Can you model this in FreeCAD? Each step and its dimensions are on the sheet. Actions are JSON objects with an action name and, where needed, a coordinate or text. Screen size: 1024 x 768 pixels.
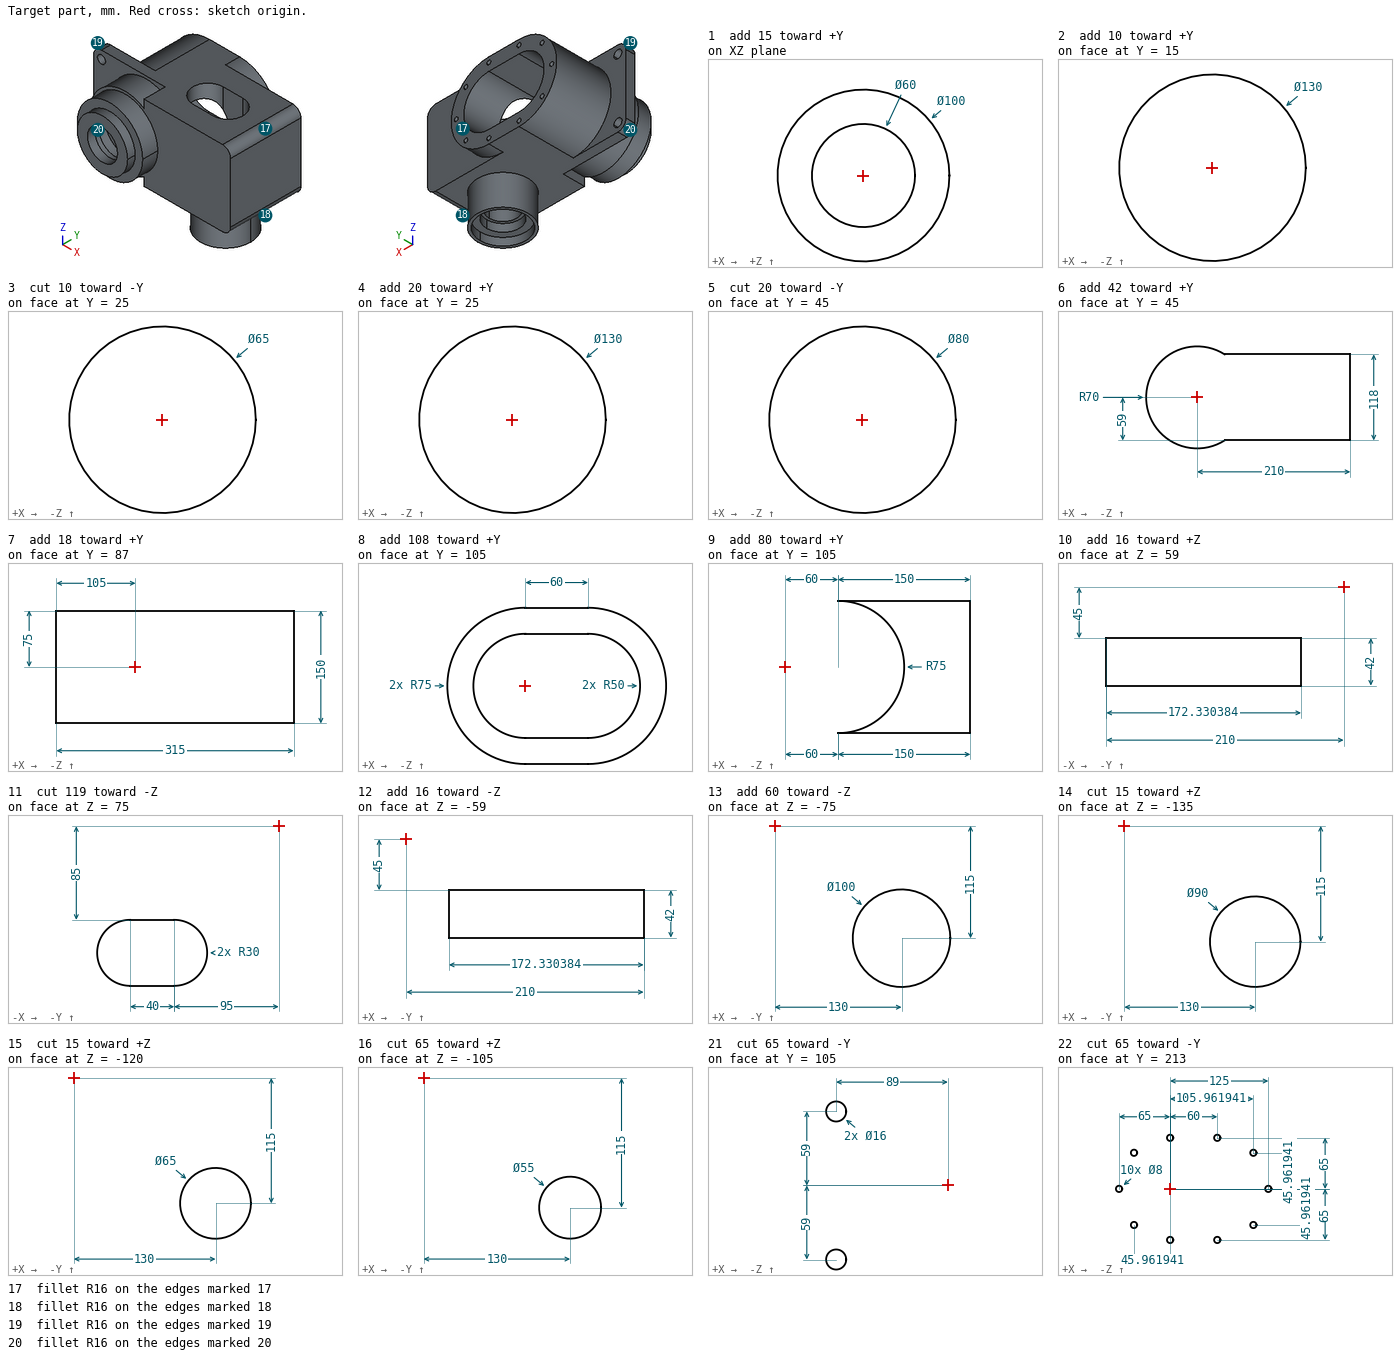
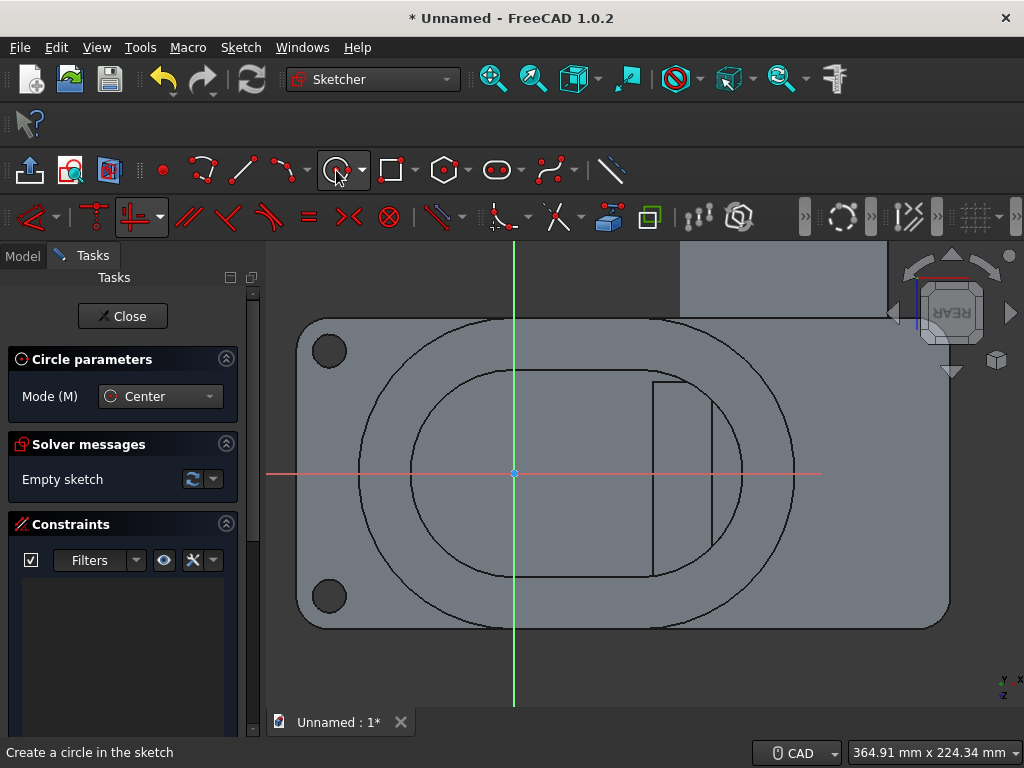
{"action": "scroll", "coordinate": [379, 474], "scroll_direction": "up", "scroll_amount": 6}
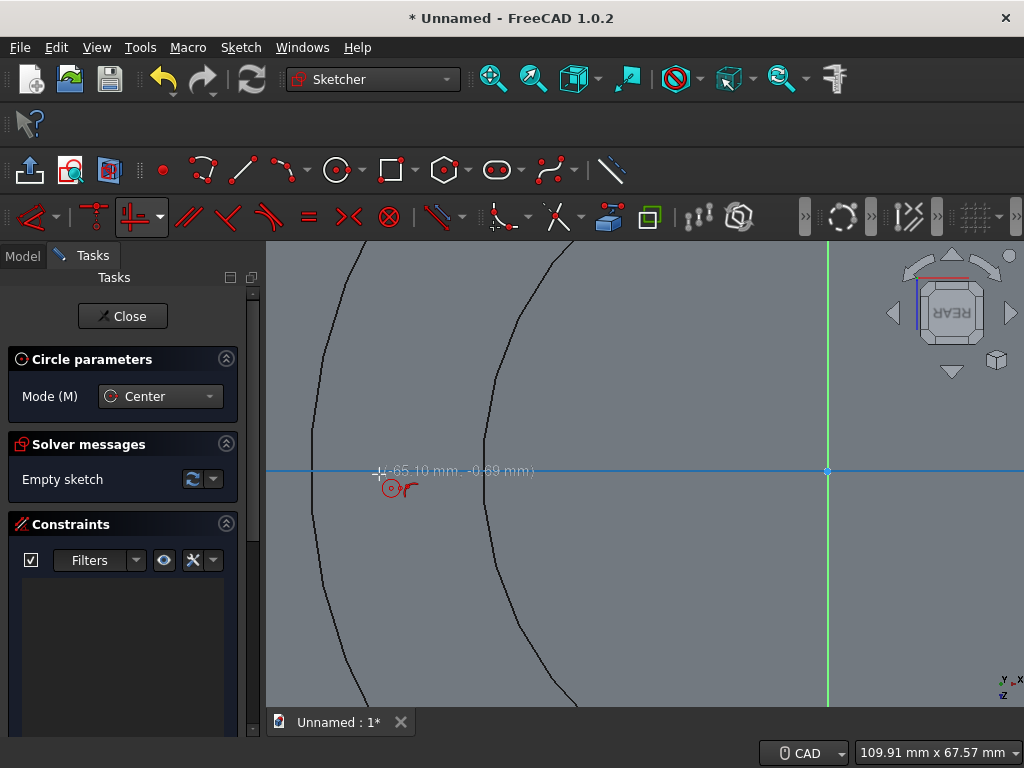
{"action": "left_click", "coordinate": [379, 471]}
{"action": "mouse_move", "coordinate": [399, 452]}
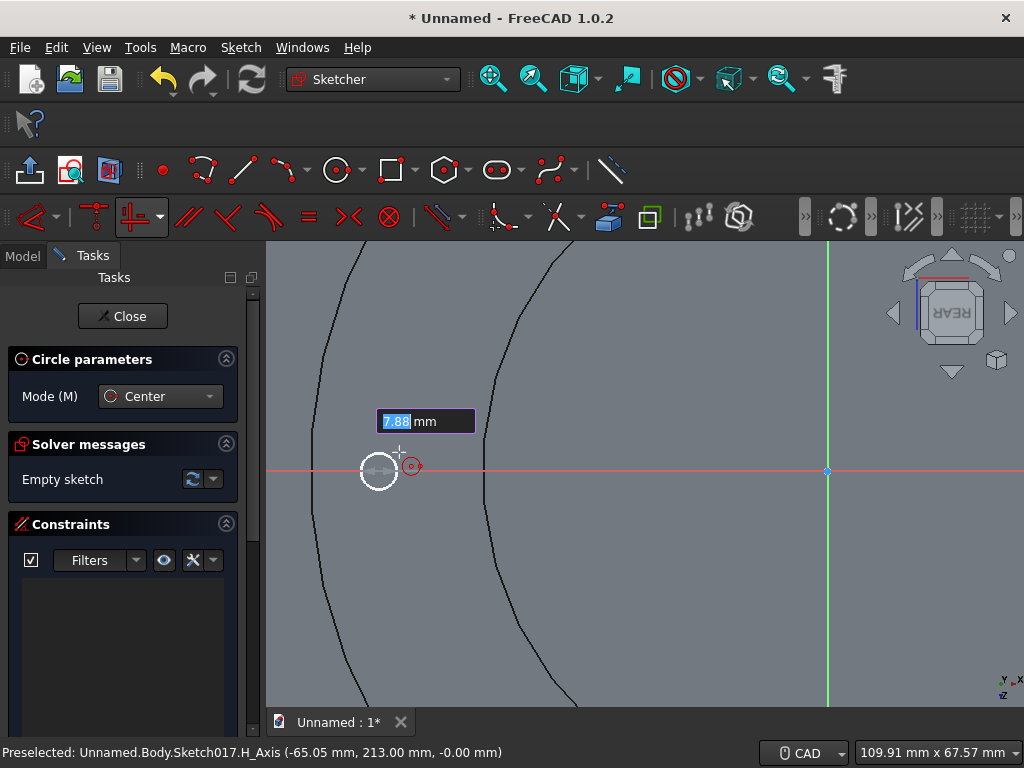
{"action": "type", "text": "8"}
{"action": "key", "text": "Return"}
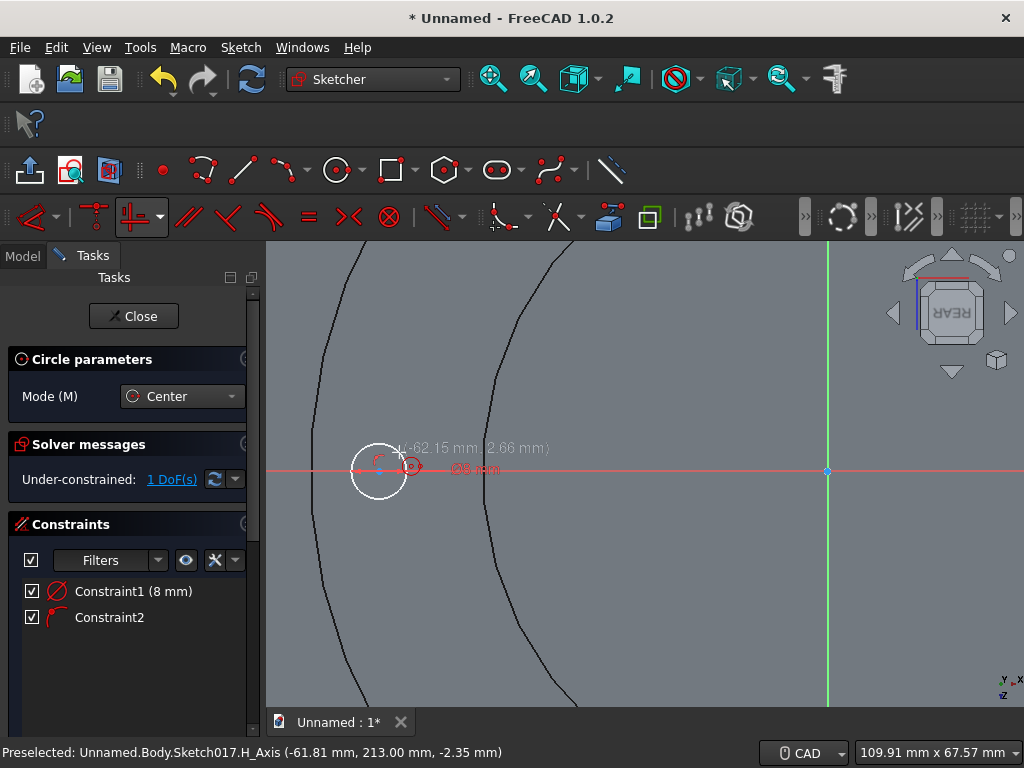
{"action": "scroll", "coordinate": [379, 475], "scroll_direction": "down", "scroll_amount": 6}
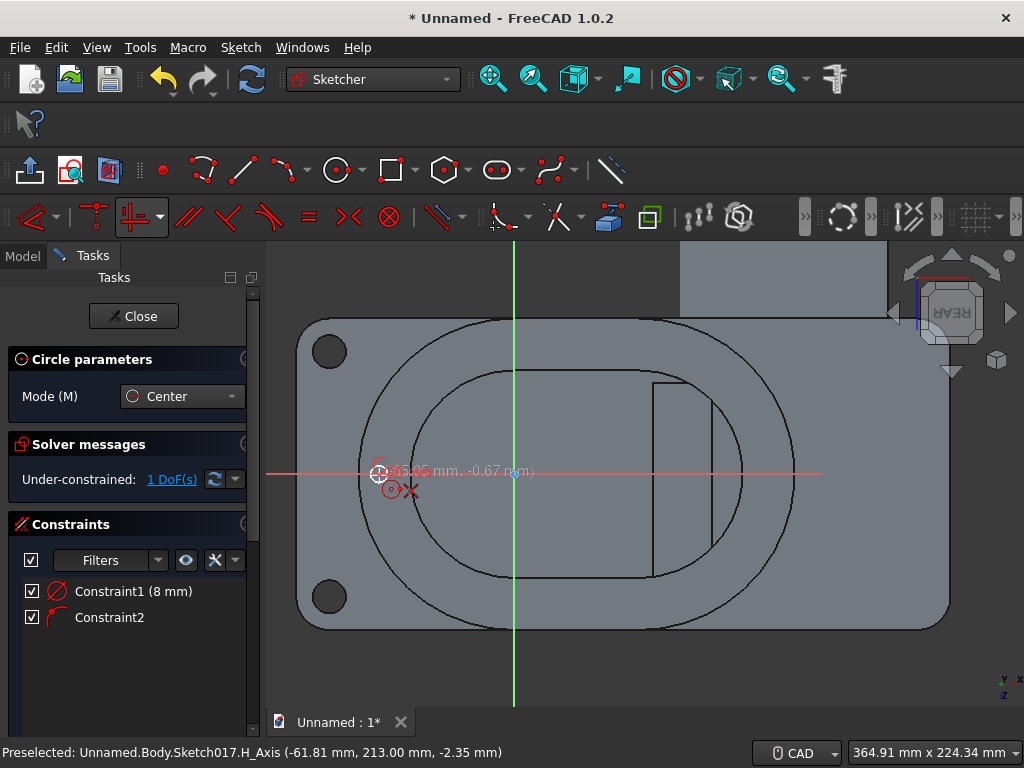
{"action": "scroll", "coordinate": [639, 339], "scroll_direction": "up", "scroll_amount": 6}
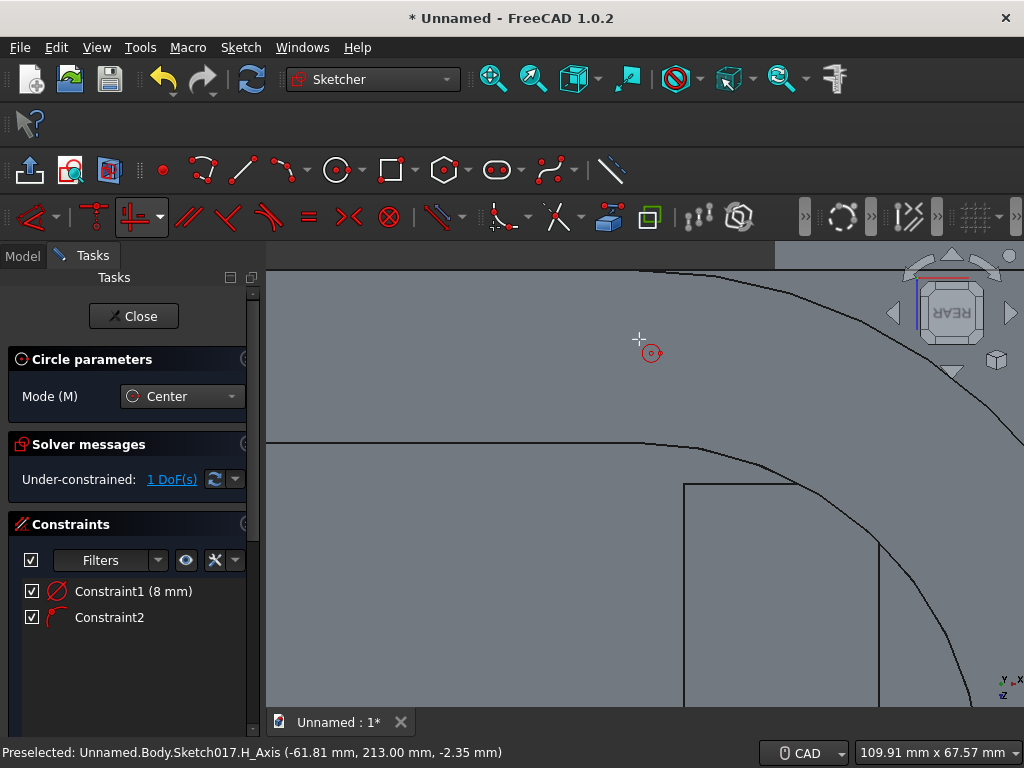
{"action": "left_click", "coordinate": [637, 339]}
{"action": "mouse_move", "coordinate": [657, 320]}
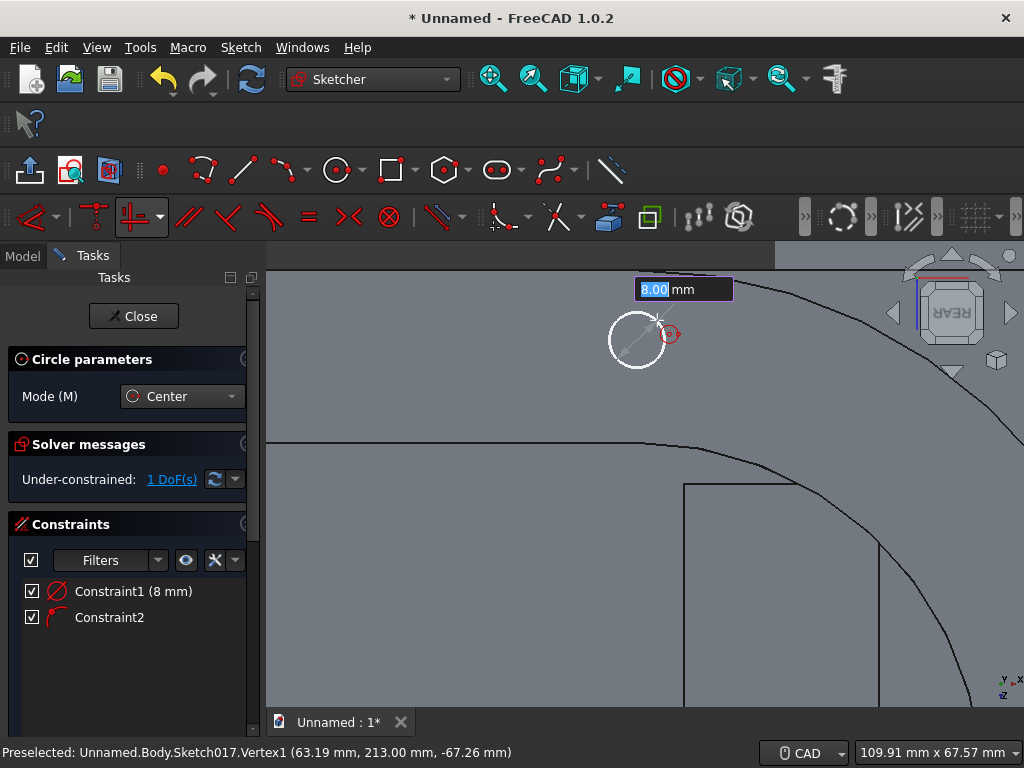
{"action": "type", "text": "8"}
{"action": "key", "text": "Return"}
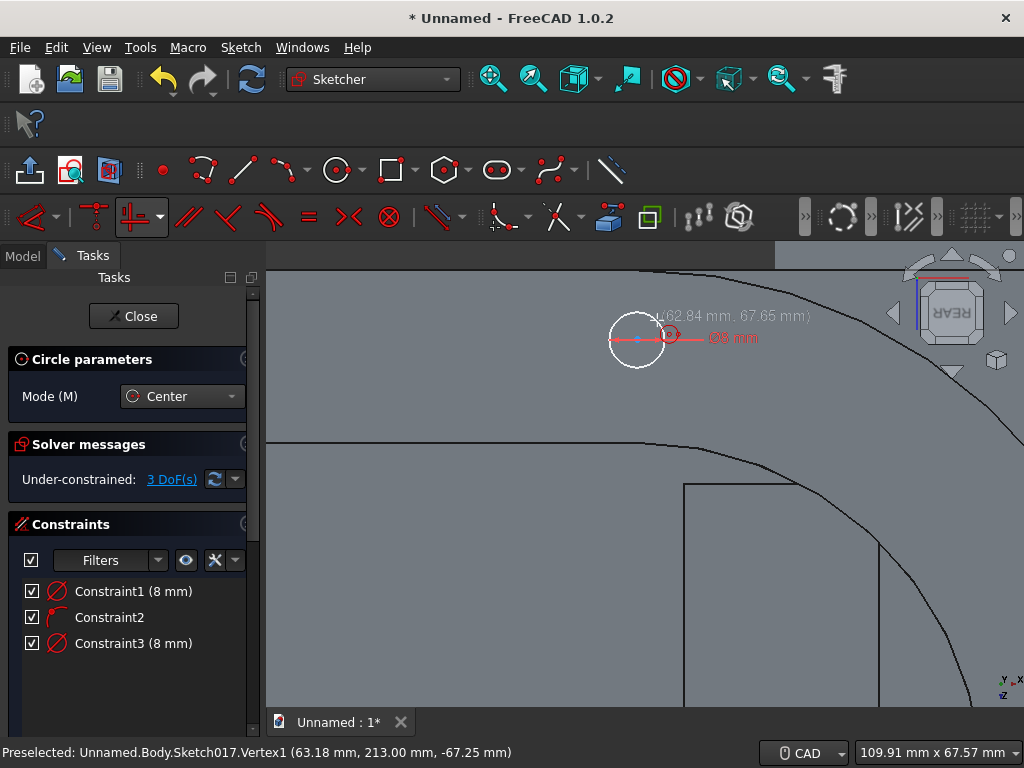
{"action": "scroll", "coordinate": [639, 339], "scroll_direction": "down", "scroll_amount": 6}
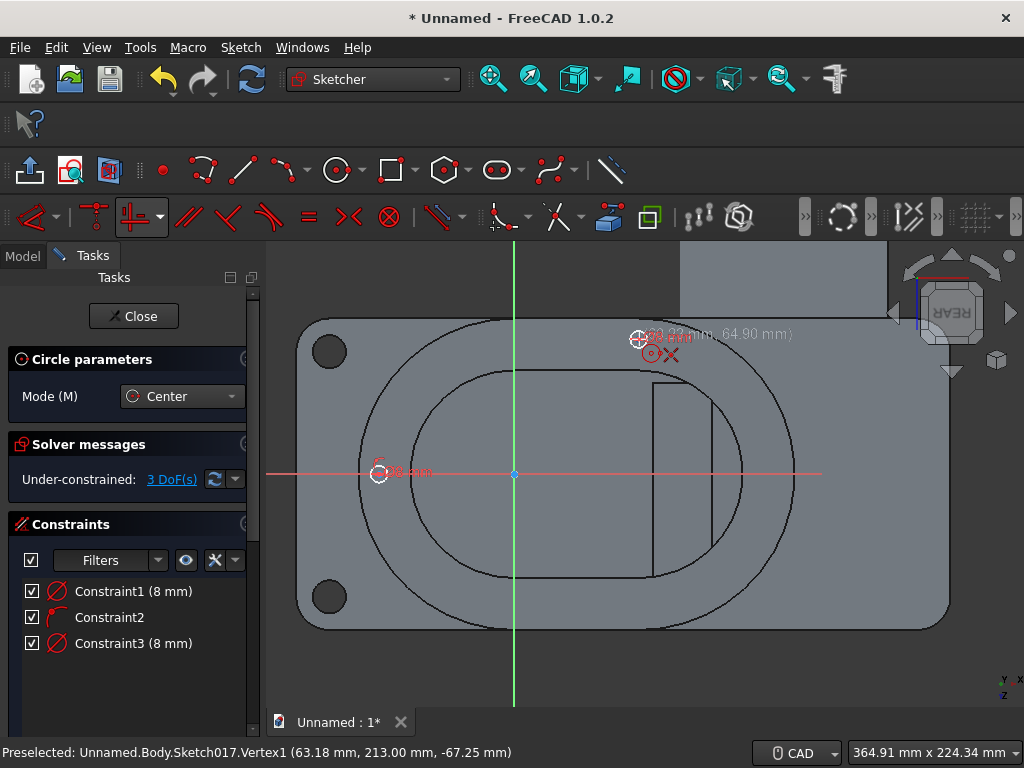
{"action": "scroll", "coordinate": [734, 379], "scroll_direction": "up", "scroll_amount": 6}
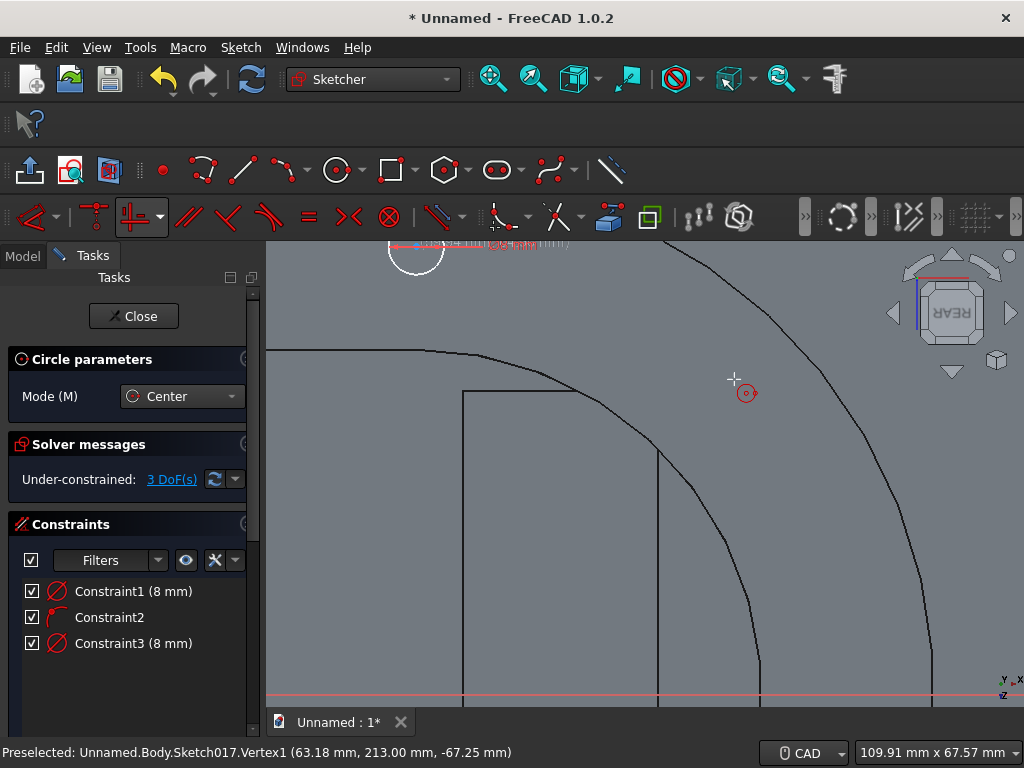
{"action": "left_click", "coordinate": [734, 378]}
{"action": "mouse_move", "coordinate": [753, 358]}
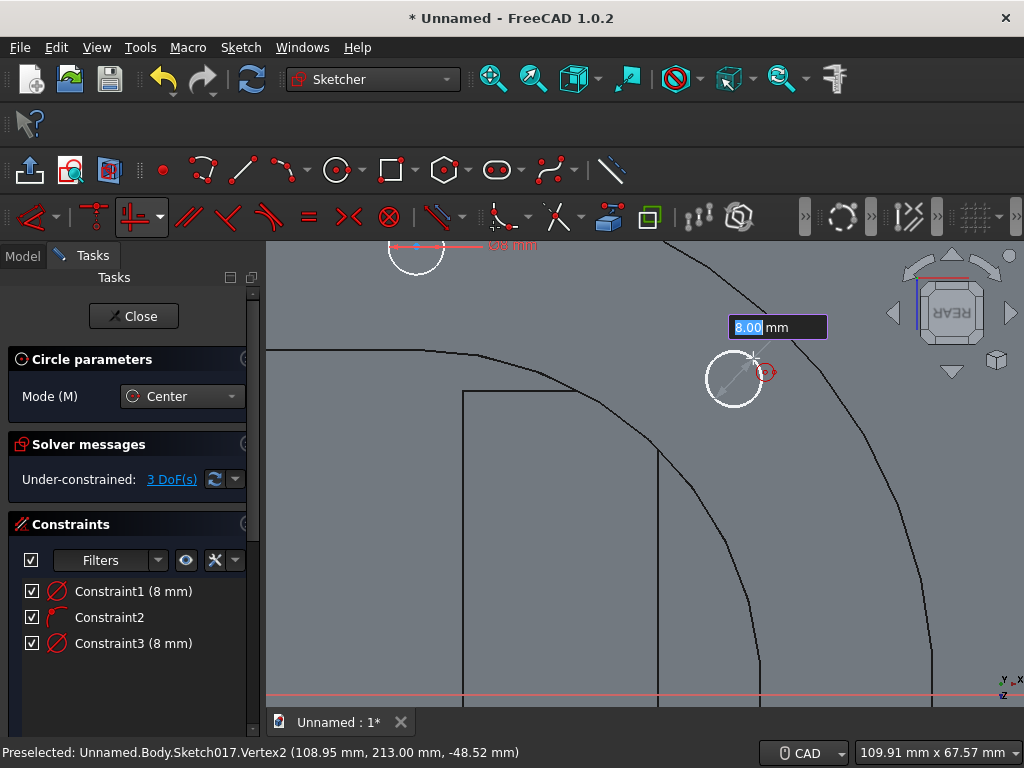
{"action": "type", "text": "8"}
{"action": "key", "text": "Return"}